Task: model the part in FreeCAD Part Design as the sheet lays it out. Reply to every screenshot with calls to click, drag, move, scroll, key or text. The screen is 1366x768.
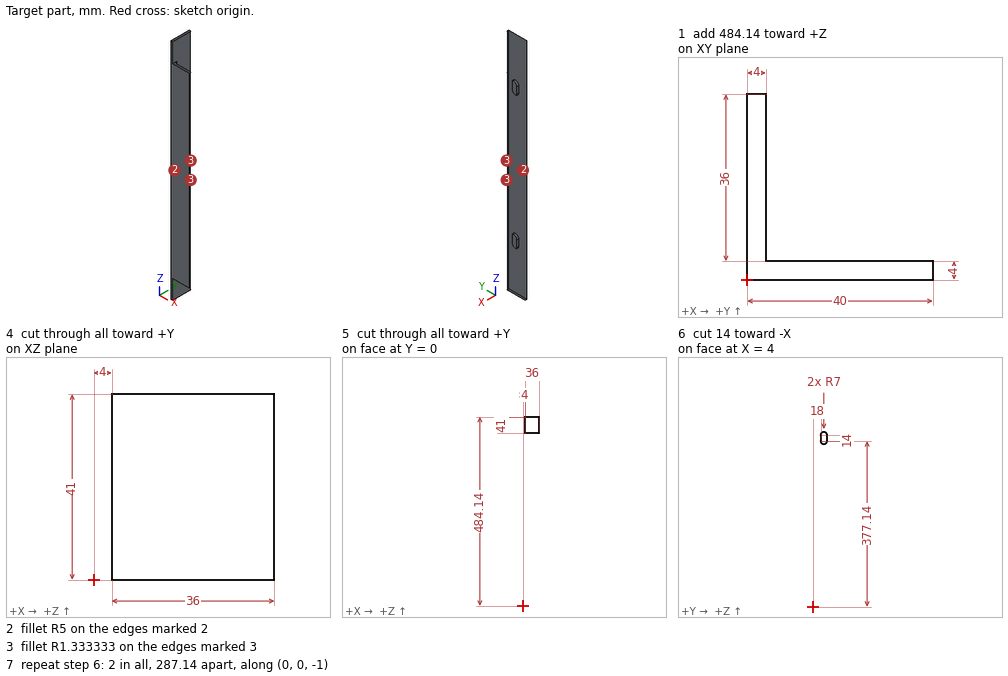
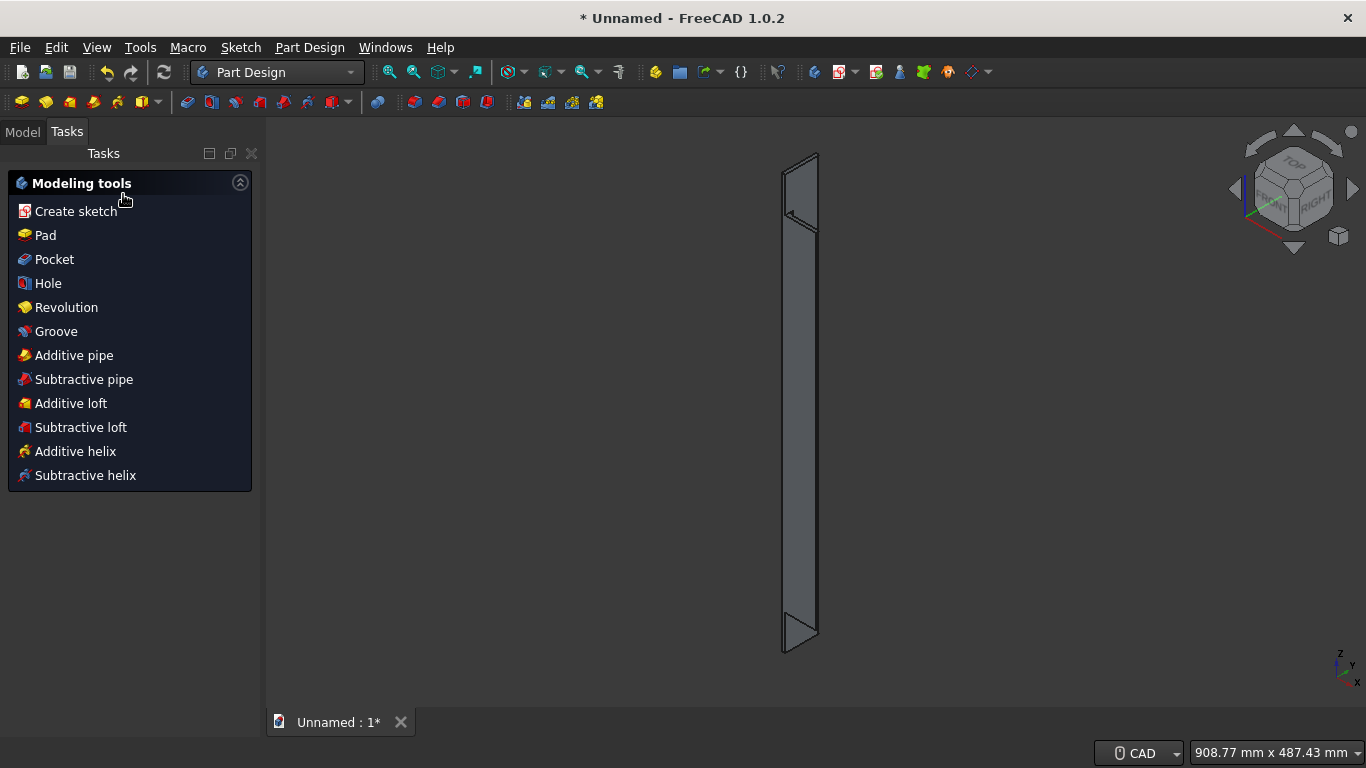
click(188, 102)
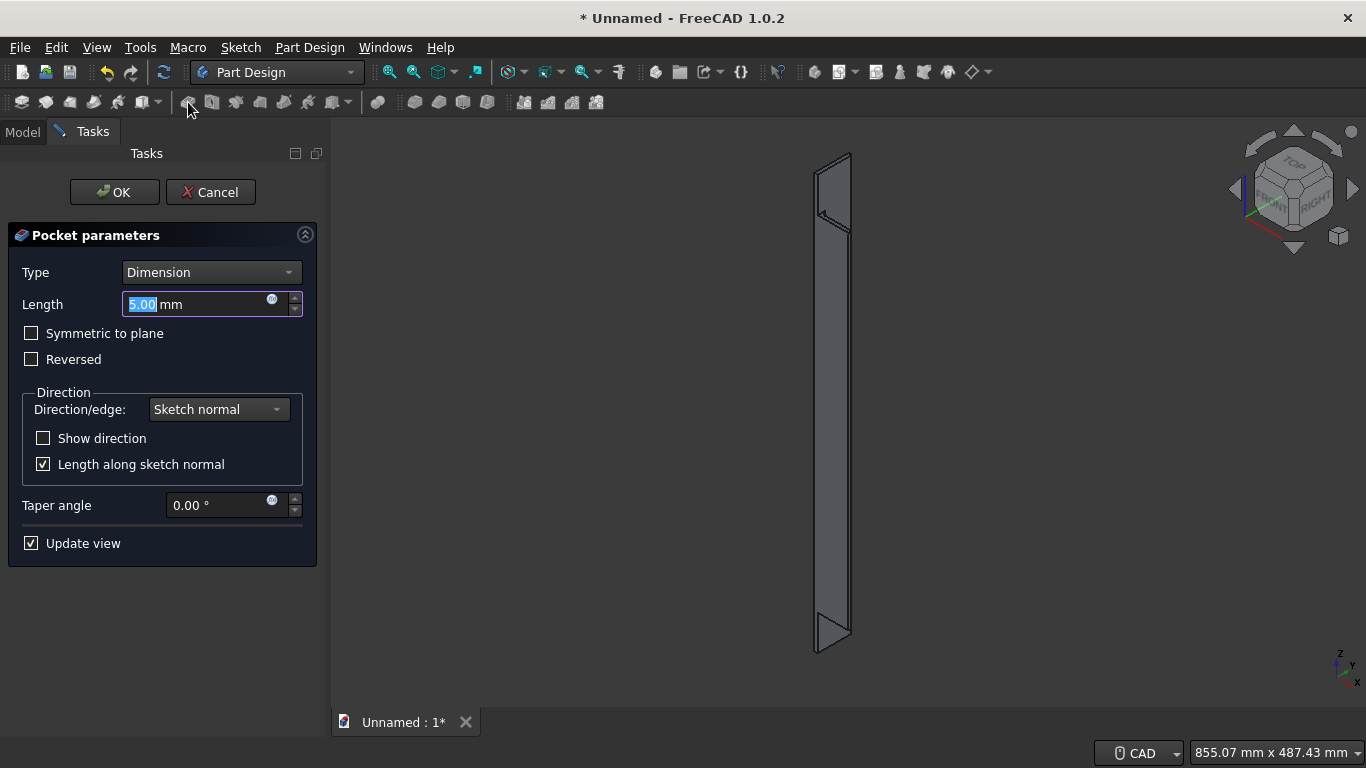
text(14)
key(Tab)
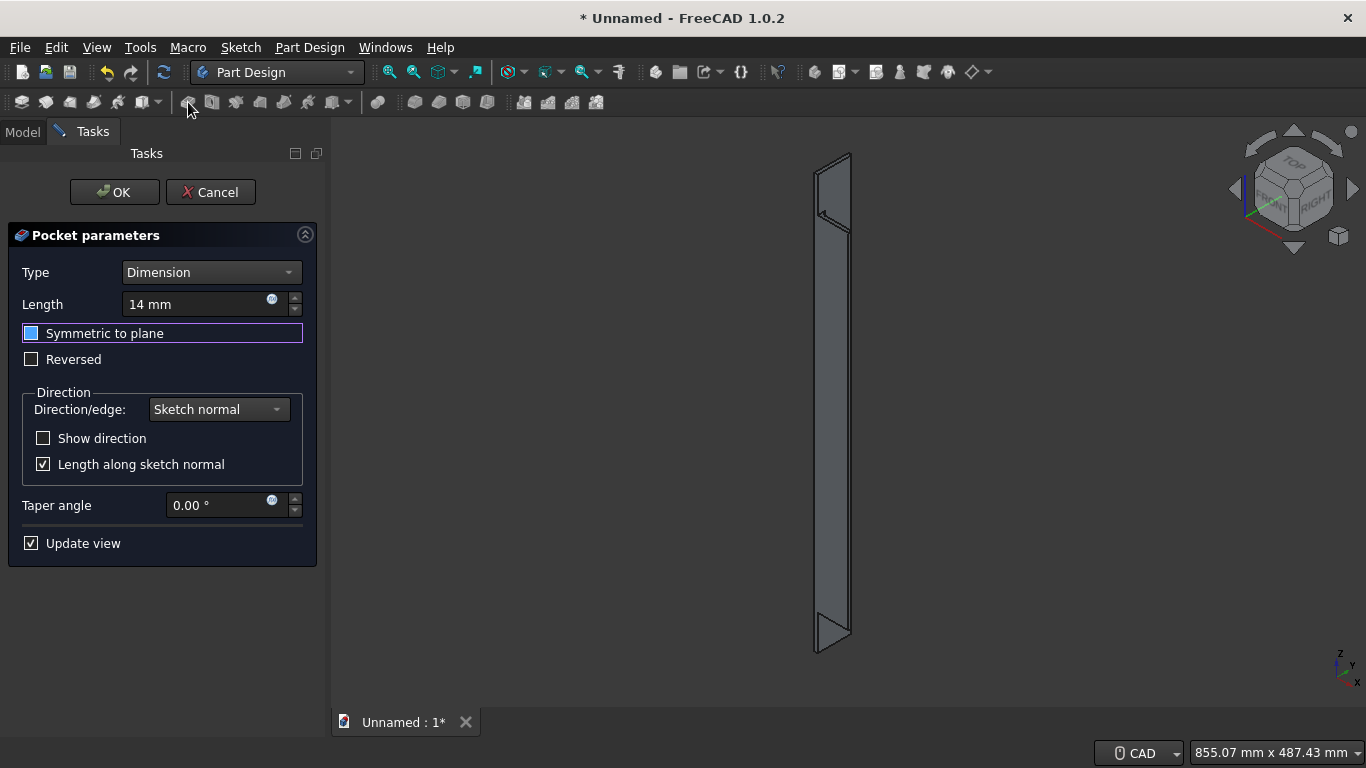
click(115, 192)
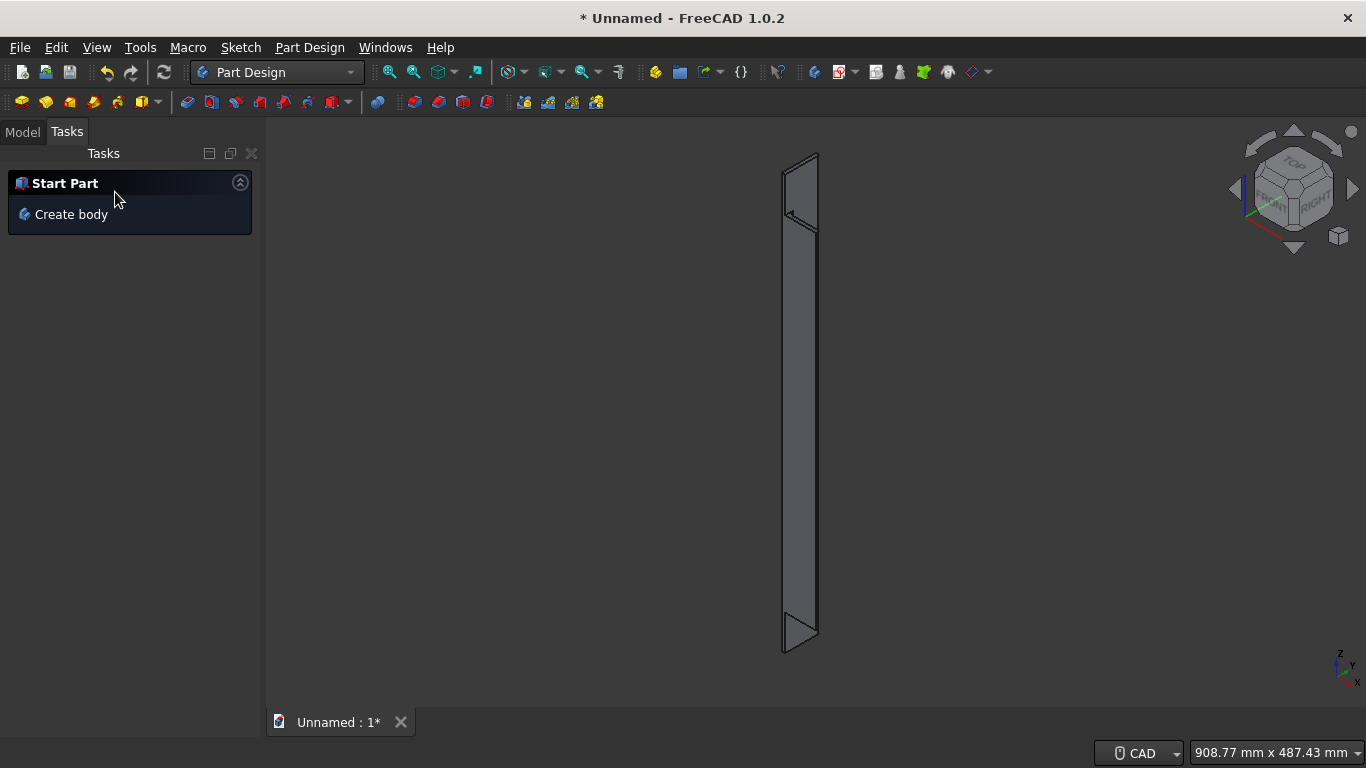
click(23, 131)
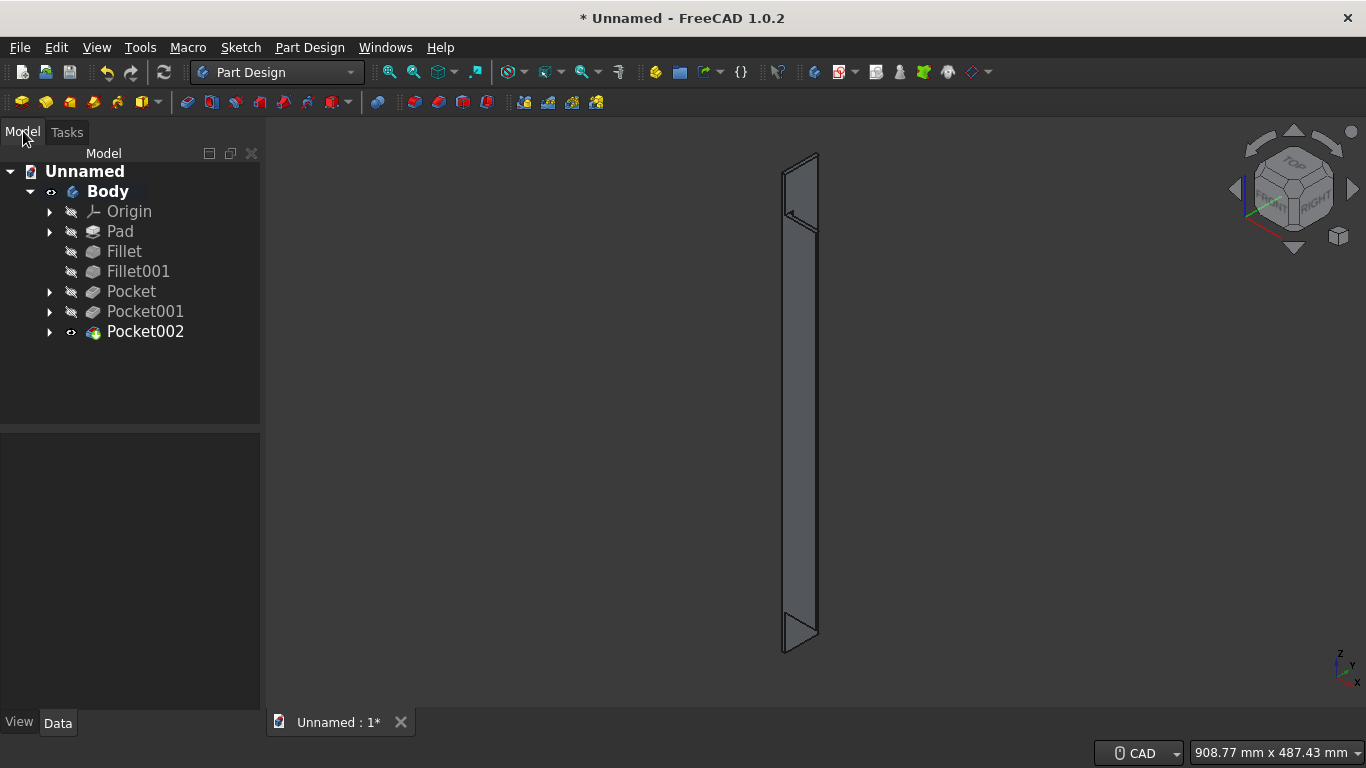
click(116, 332)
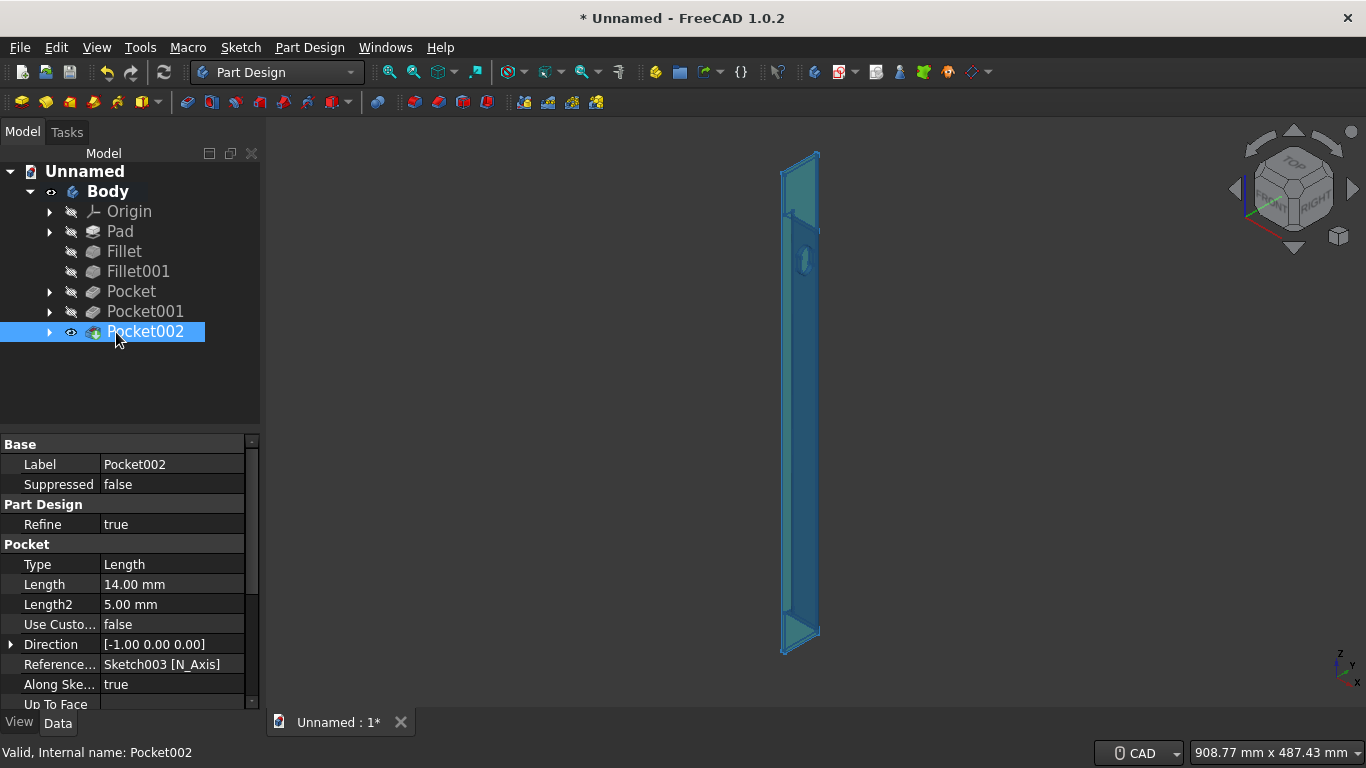
click(548, 102)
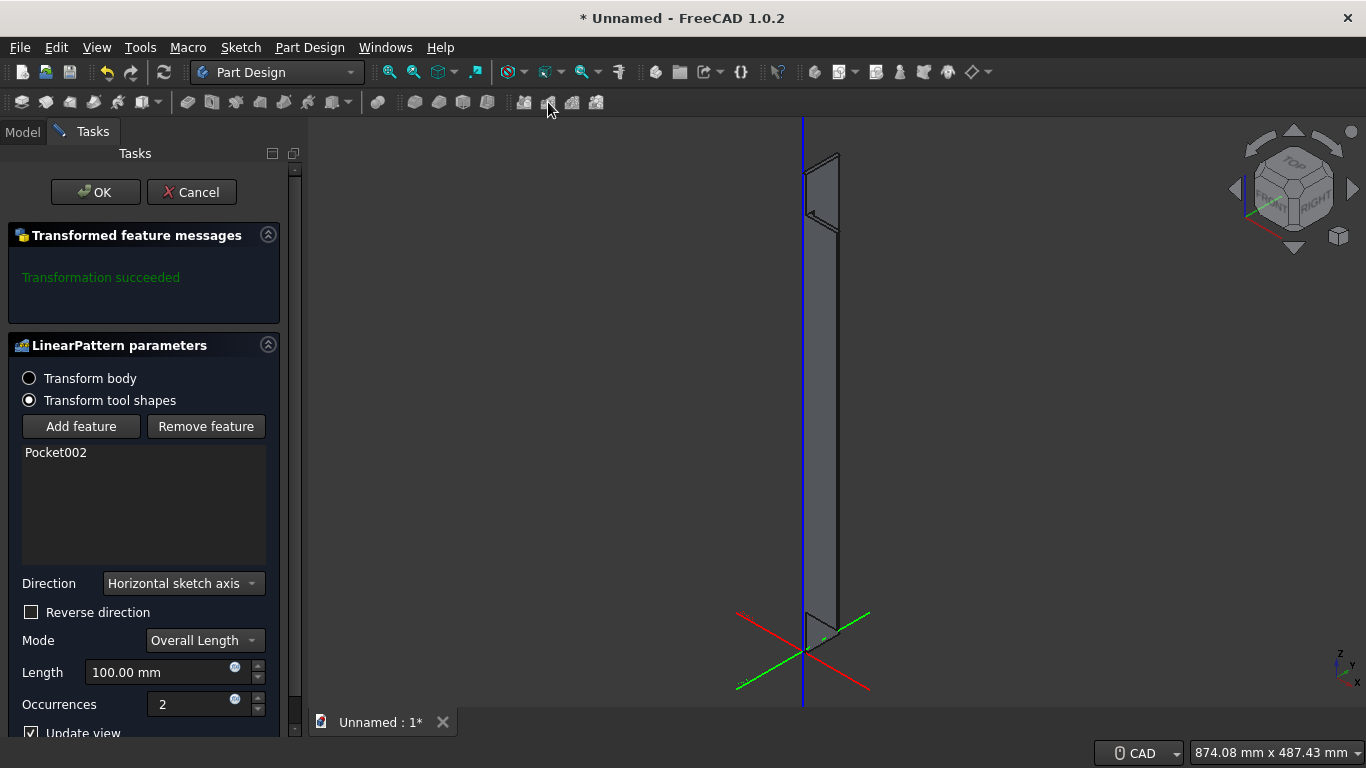
click(184, 584)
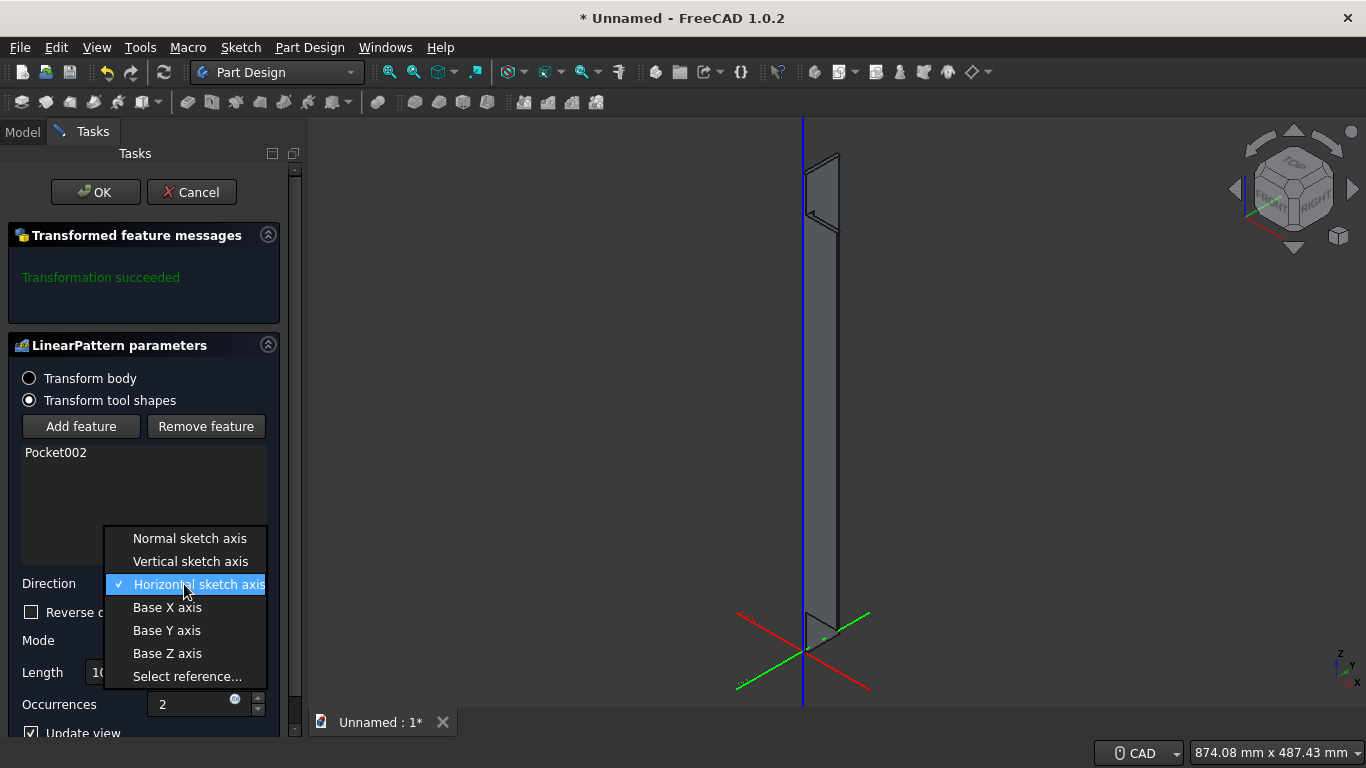
click(184, 654)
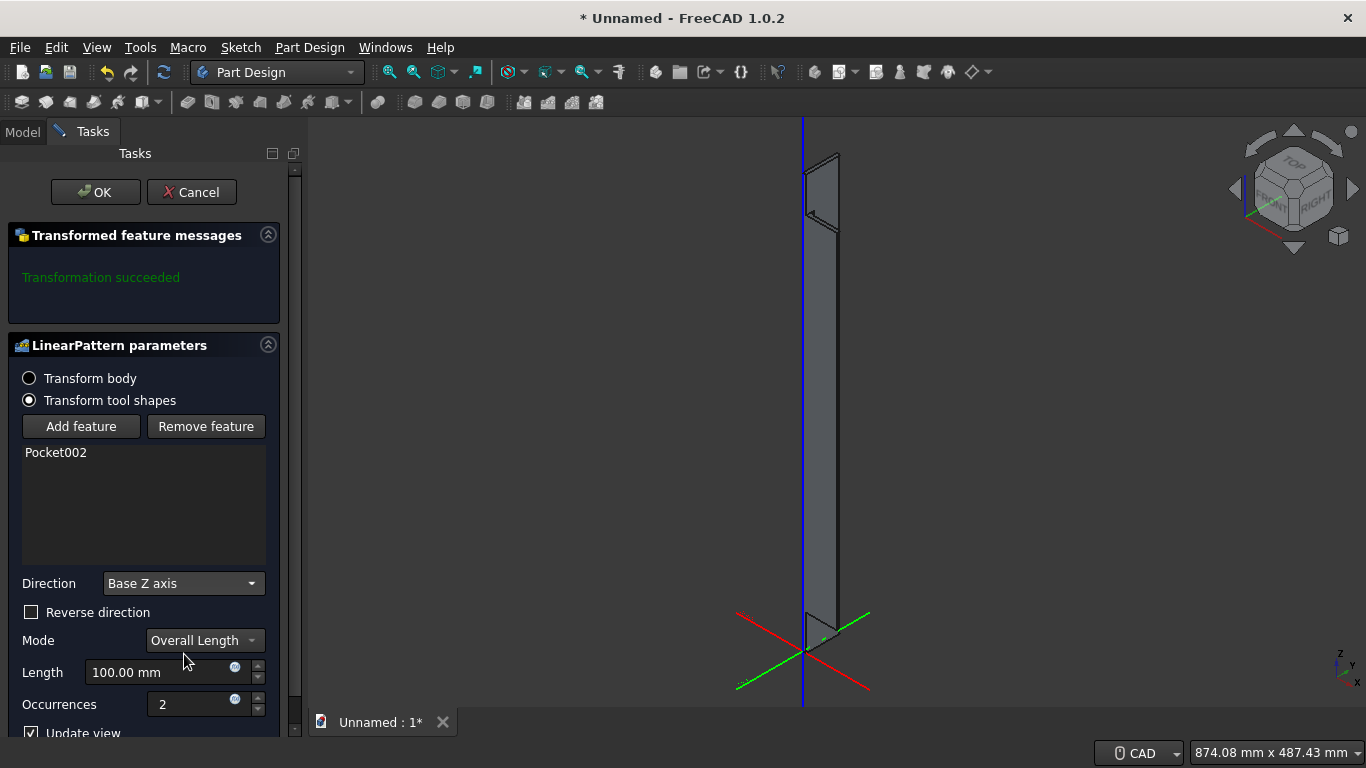
click(206, 640)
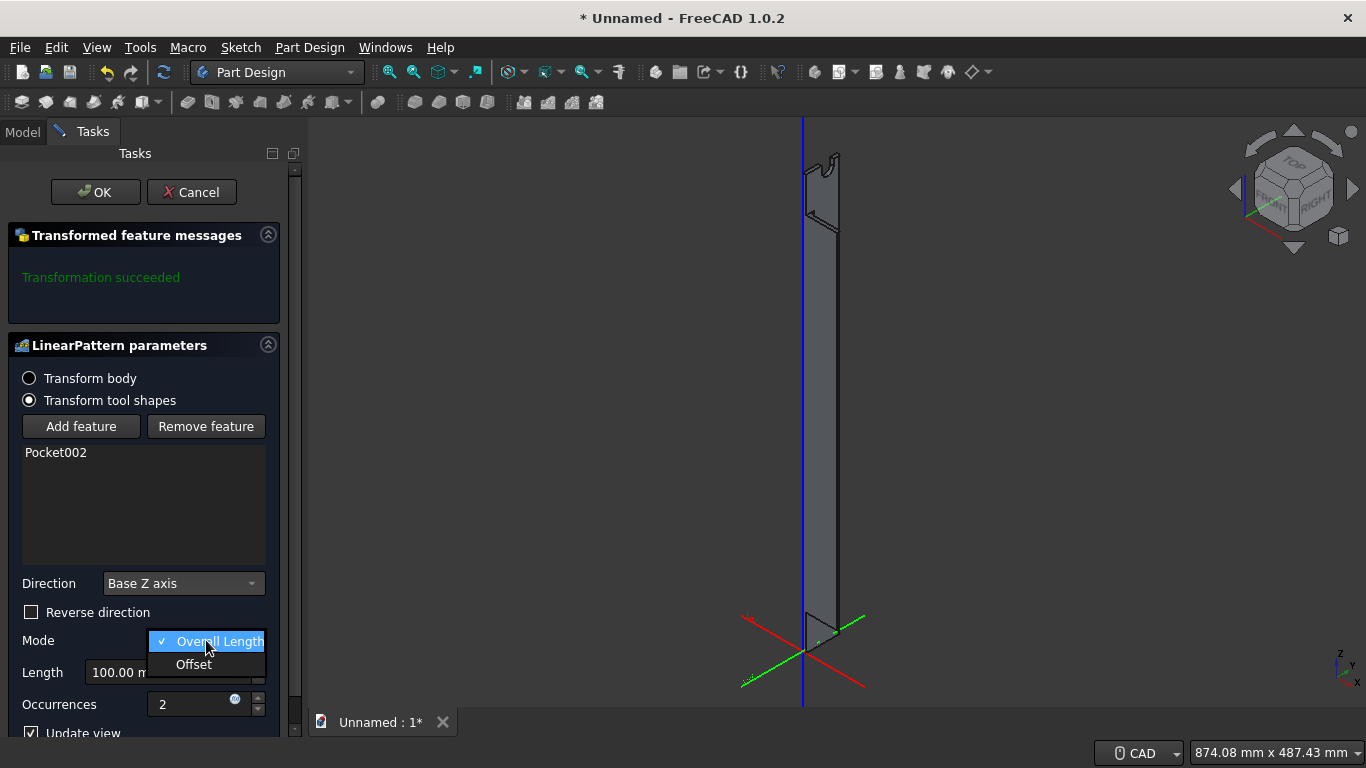
click(206, 664)